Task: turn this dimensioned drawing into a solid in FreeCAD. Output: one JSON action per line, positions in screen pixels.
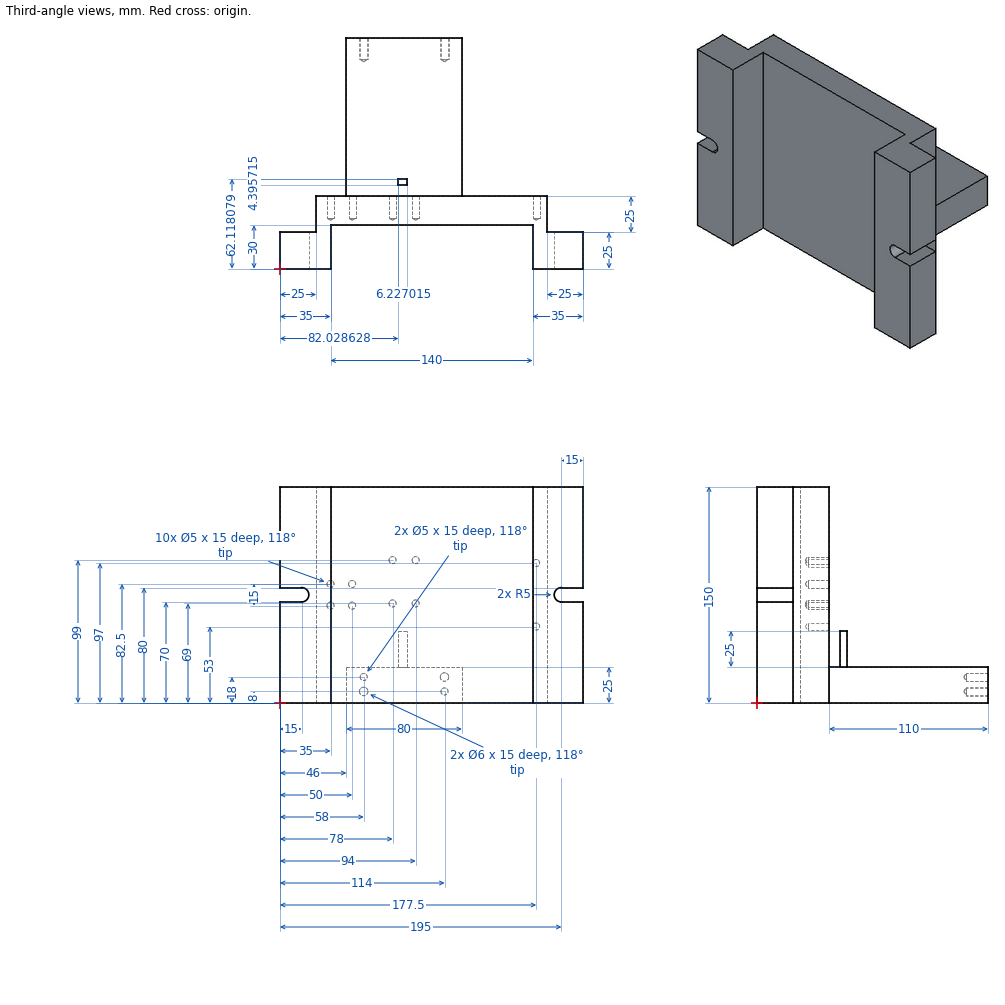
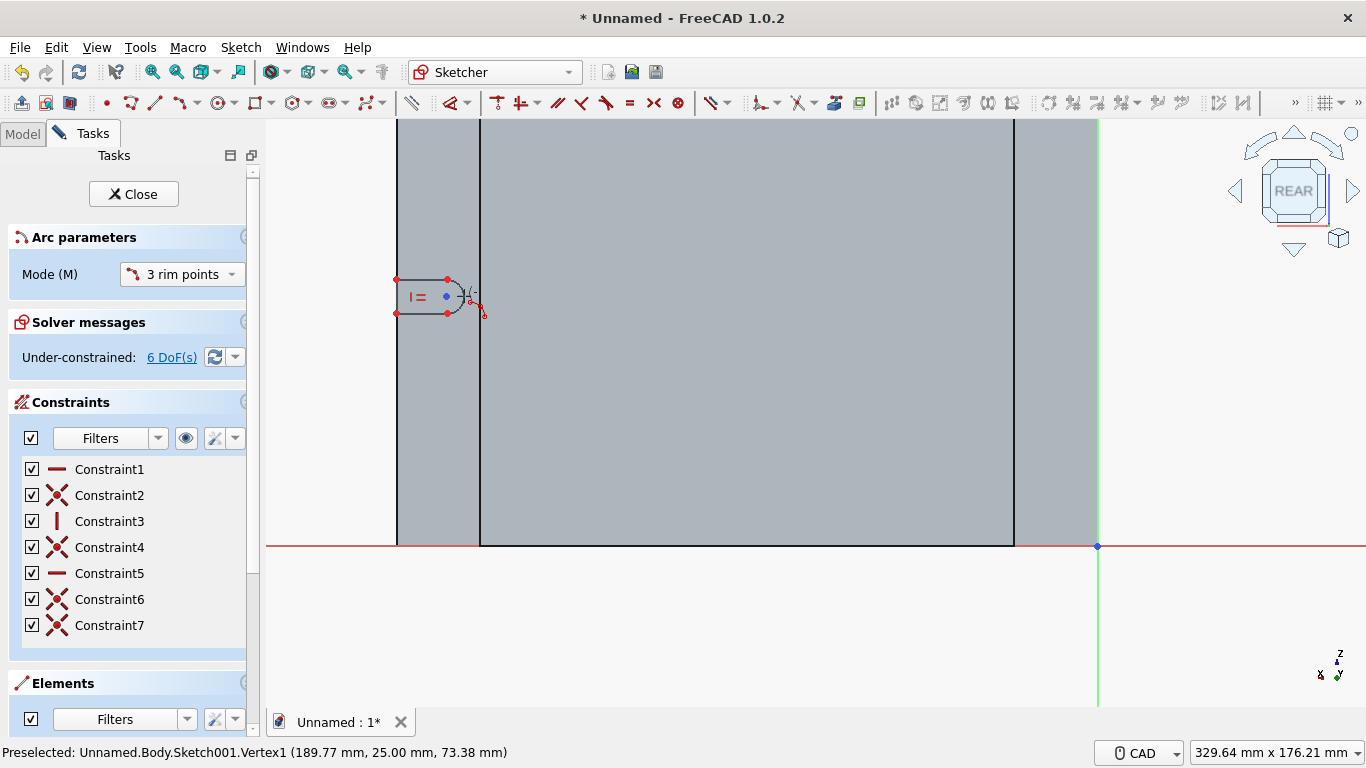
{"action": "key", "text": "g m"}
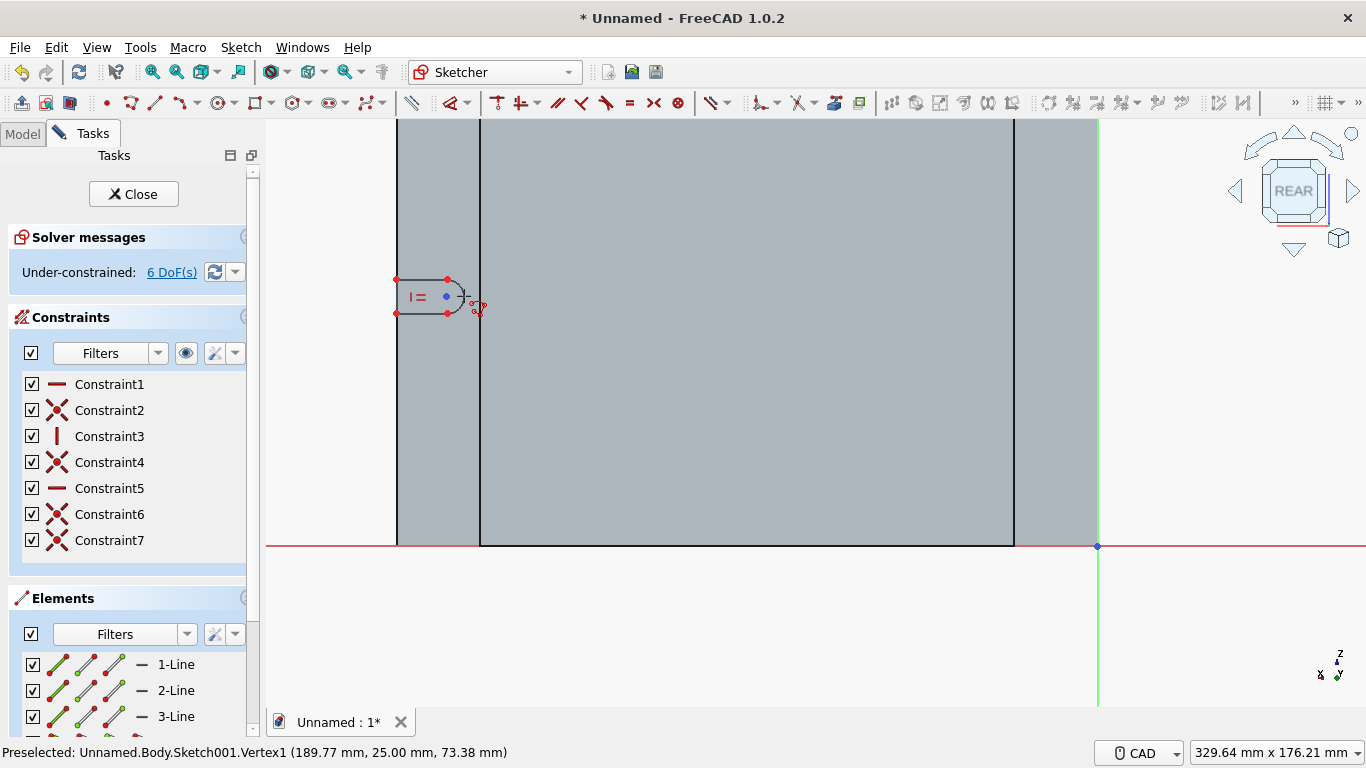
{"action": "left_click", "coordinate": [1048, 313]}
{"action": "left_click", "coordinate": [1098, 313]}
{"action": "left_click", "coordinate": [1089, 279]}
{"action": "left_click", "coordinate": [1048, 279]}
{"action": "right_click", "coordinate": [1048, 279]}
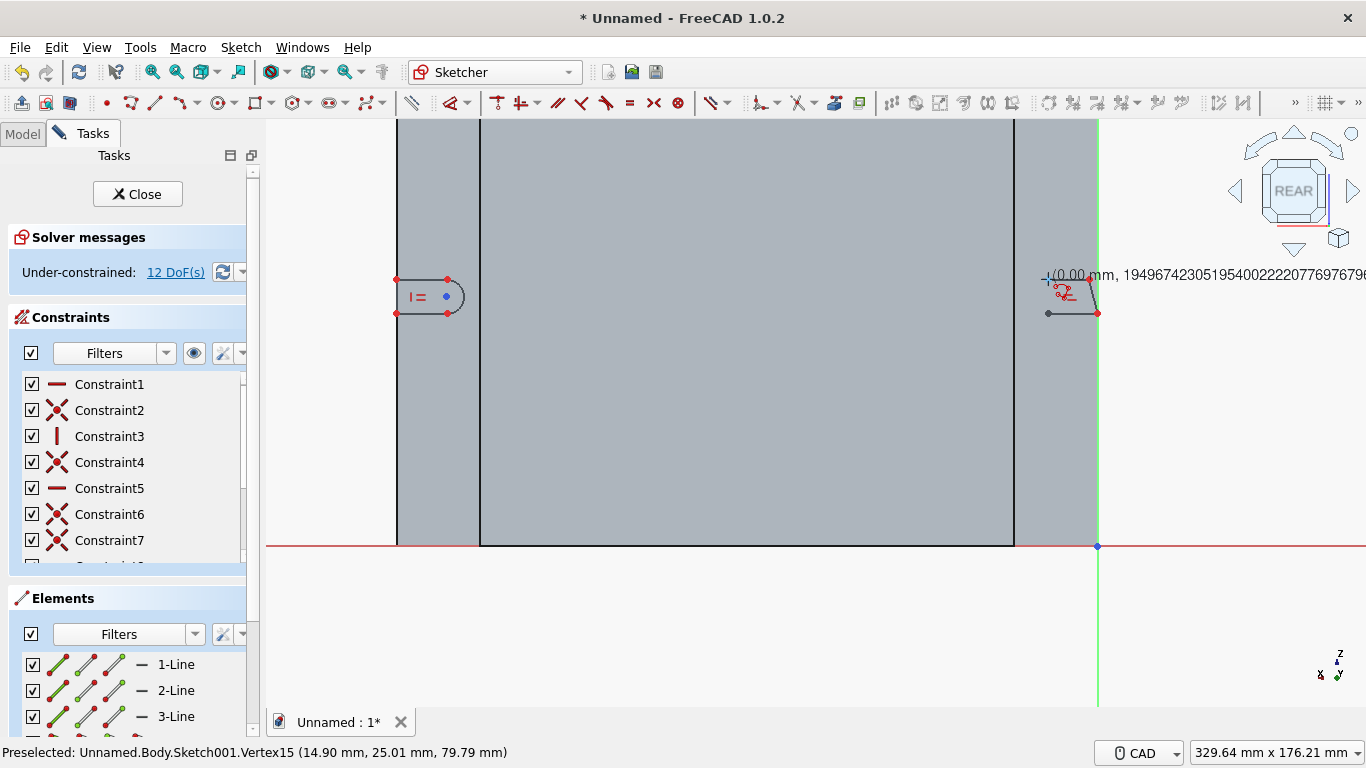
{"action": "left_click", "coordinate": [180, 104]}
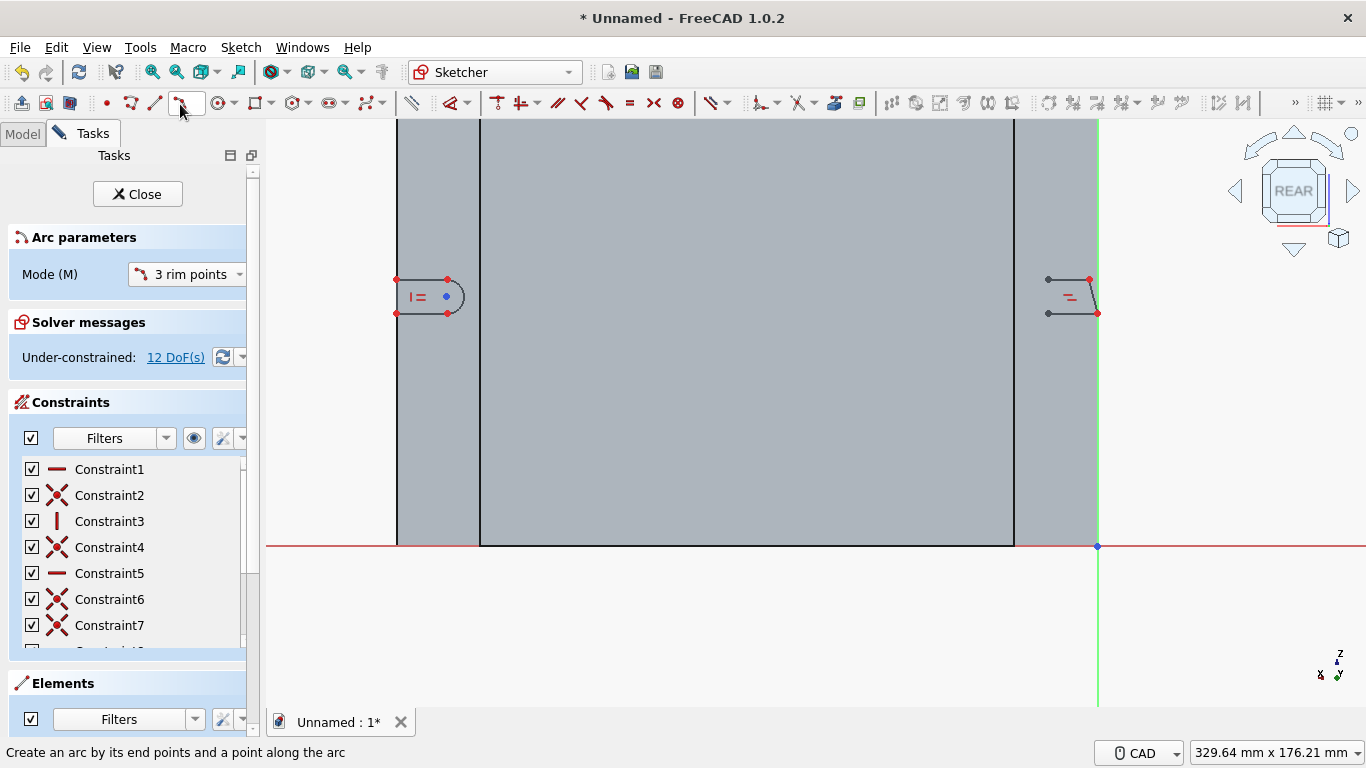
{"action": "left_click", "coordinate": [1048, 280]}
{"action": "left_click", "coordinate": [1048, 314]}
{"action": "left_click", "coordinate": [1031, 296]}
{"action": "key", "text": "Escape"}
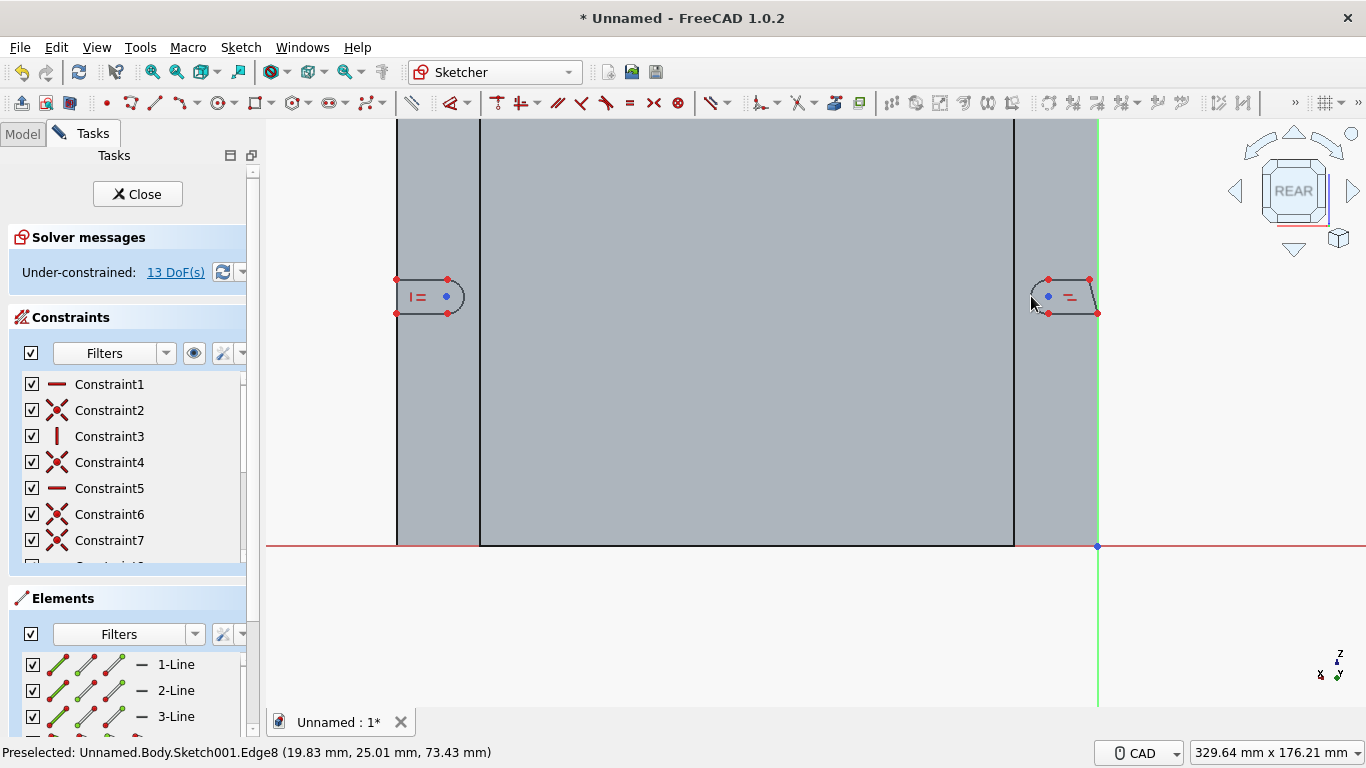
{"action": "left_click", "coordinate": [432, 280]}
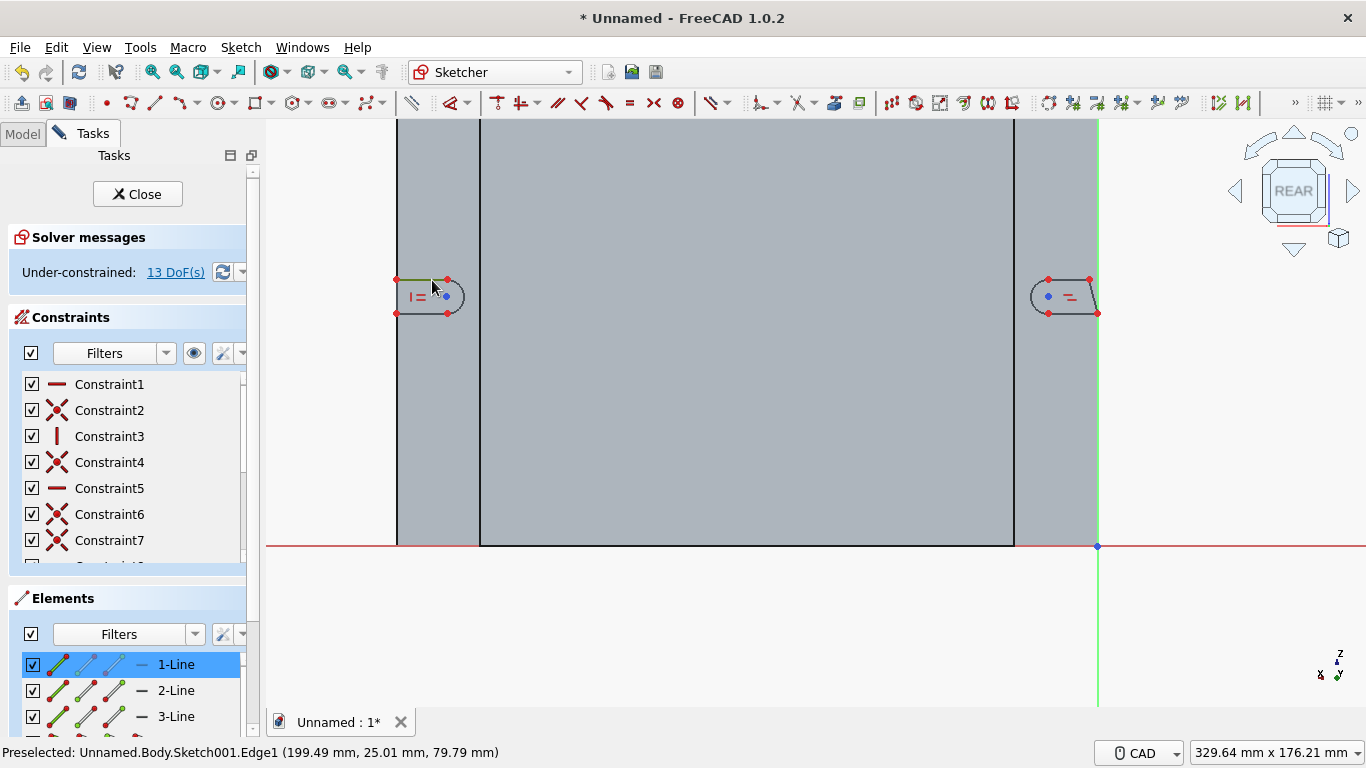
{"action": "left_click", "coordinate": [461, 307]}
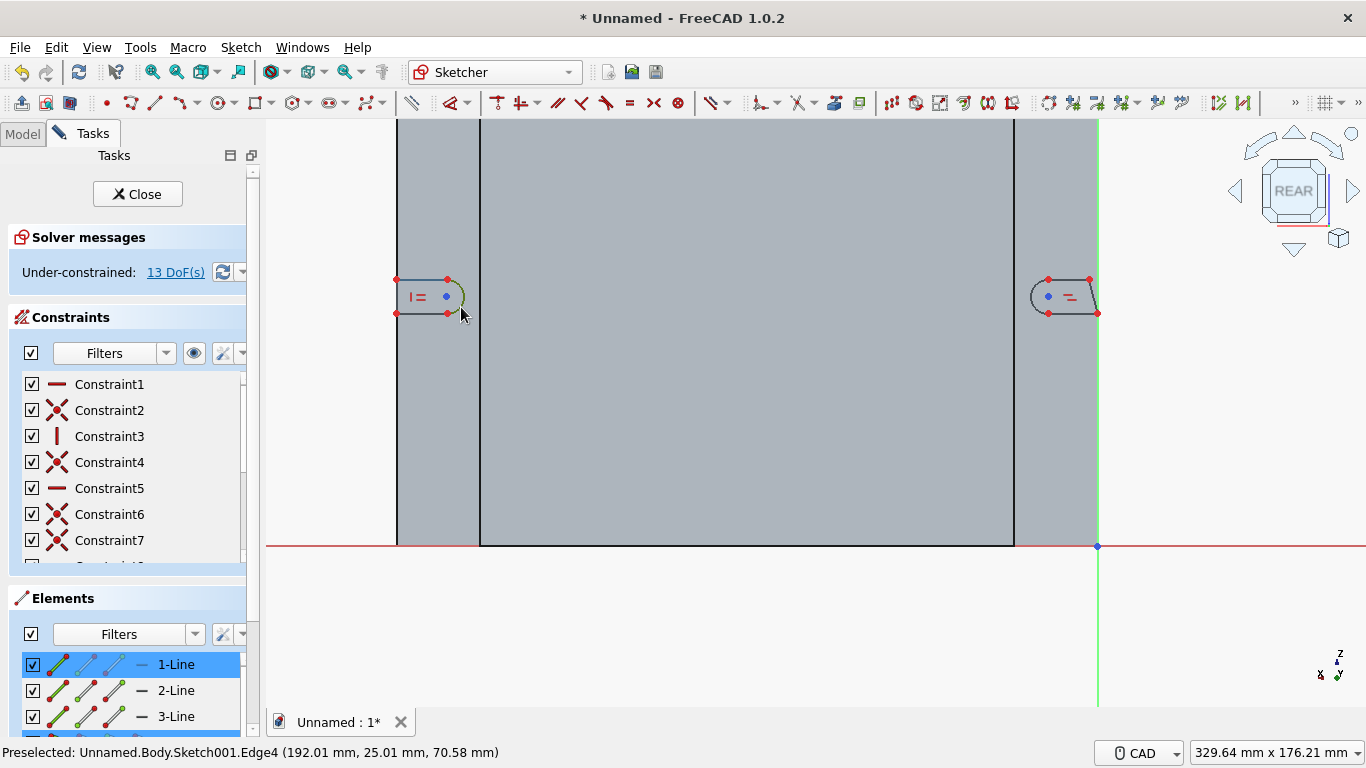
{"action": "key", "text": "t"}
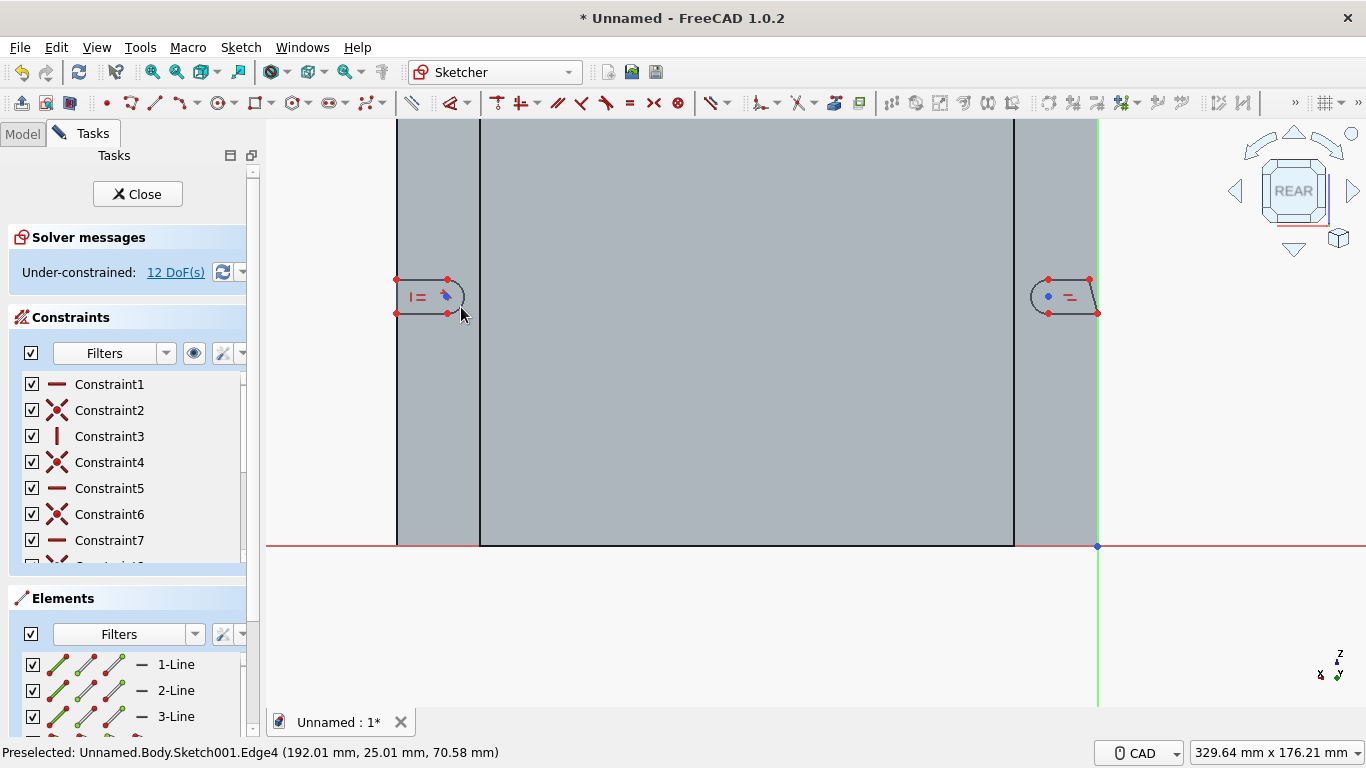
{"action": "left_click", "coordinate": [412, 314]}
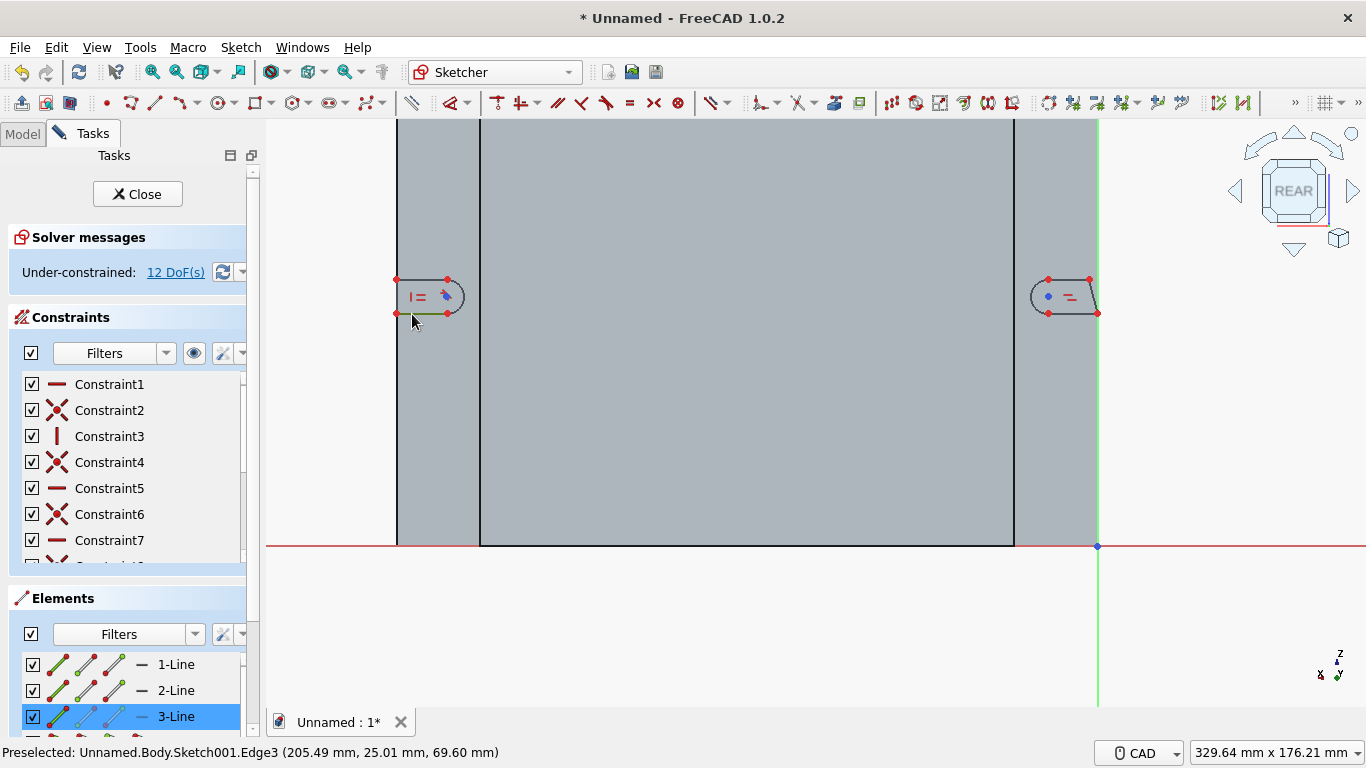
{"action": "left_click", "coordinate": [461, 307]}